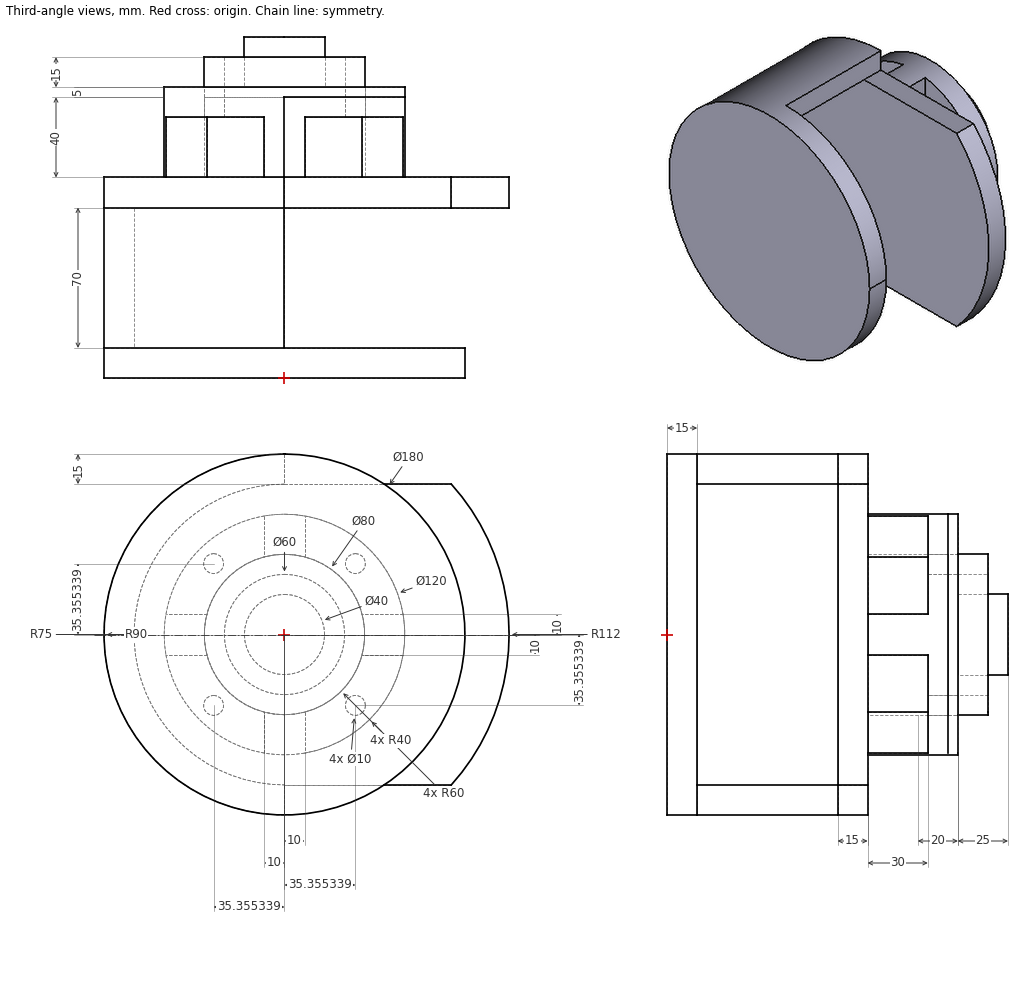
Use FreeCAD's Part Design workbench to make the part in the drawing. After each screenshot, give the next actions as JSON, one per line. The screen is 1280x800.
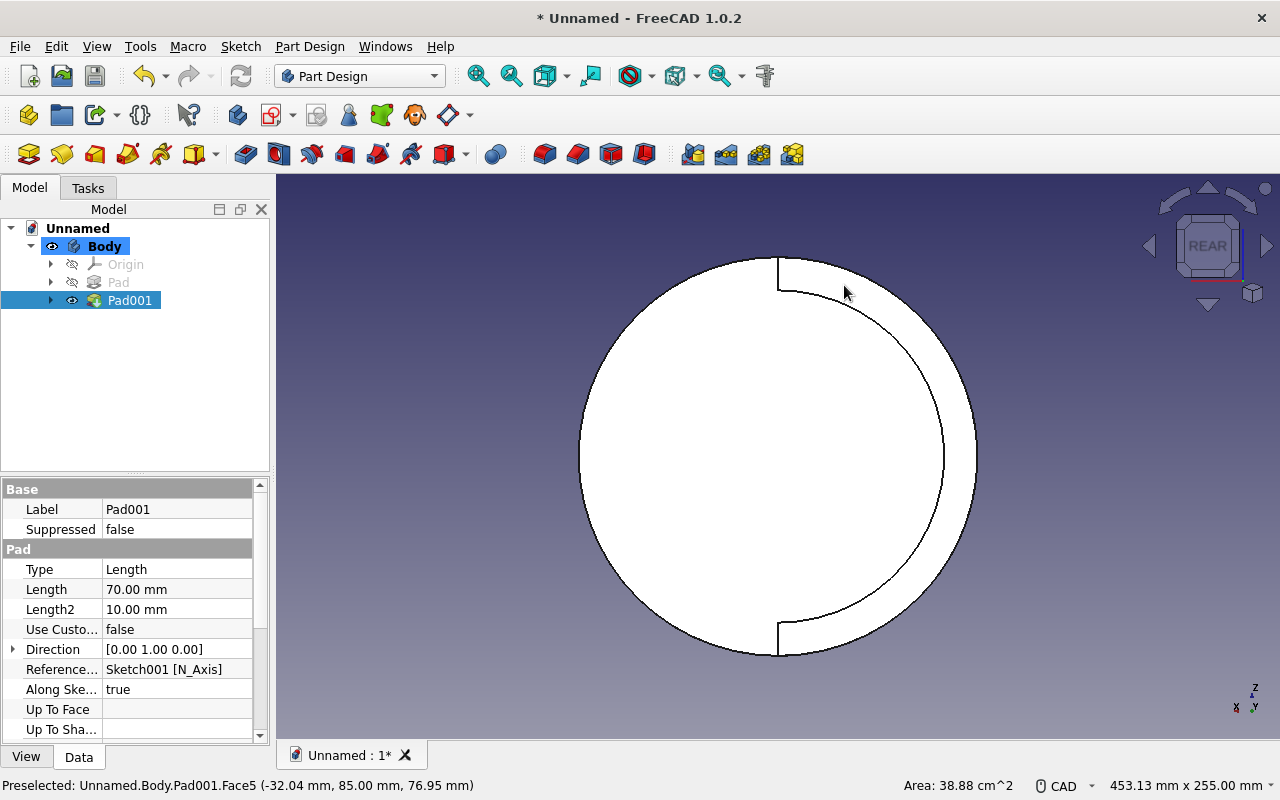
{"action": "left_click", "coordinate": [270, 116]}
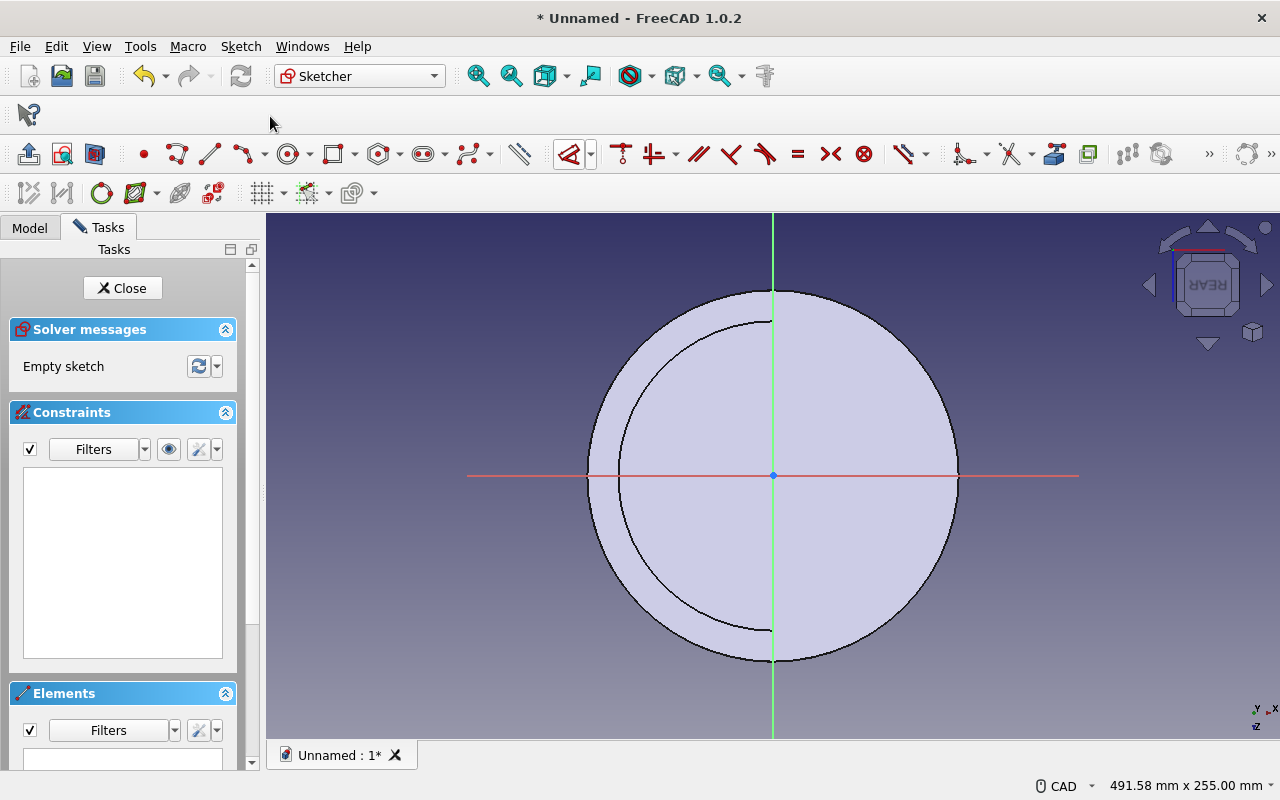
{"action": "key", "text": "g m"}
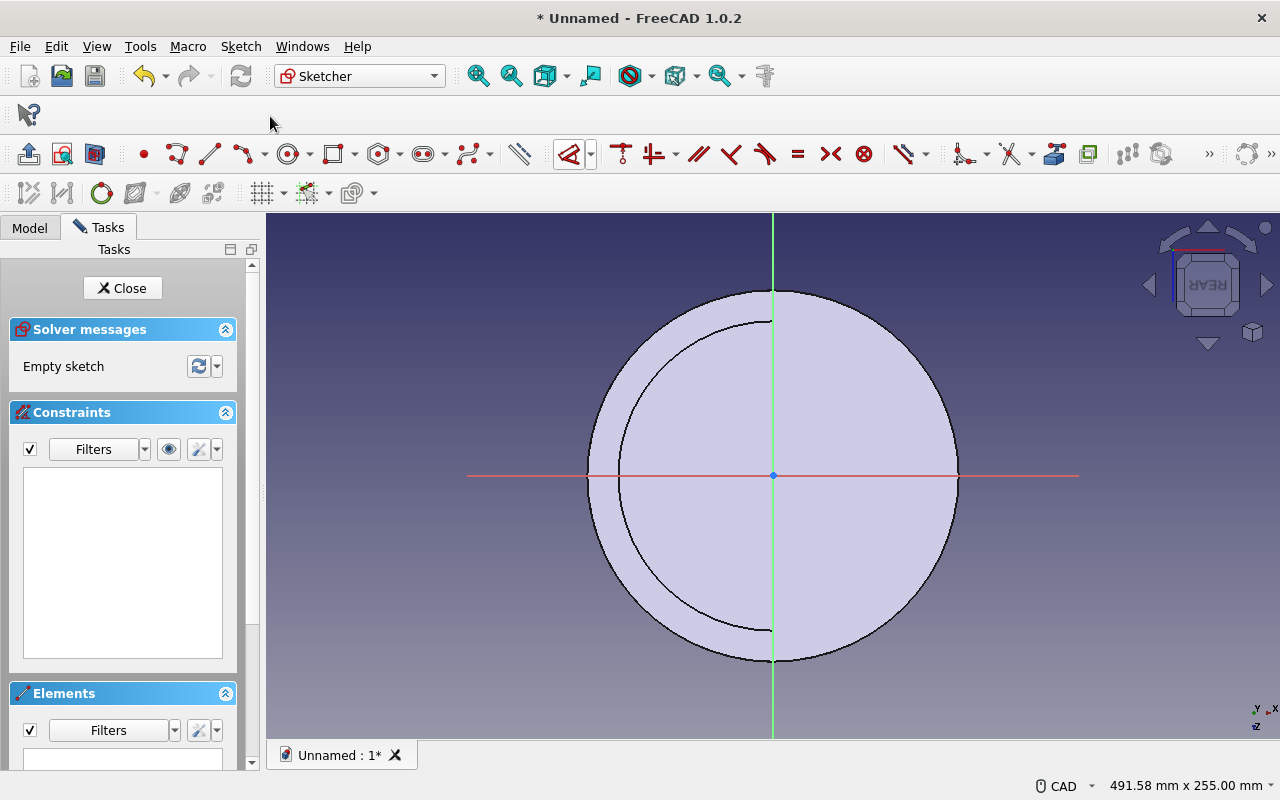
{"action": "left_click", "coordinate": [773, 662]}
{"action": "left_click", "coordinate": [782, 631]}
{"action": "left_click", "coordinate": [945, 631]}
{"action": "right_click", "coordinate": [945, 631]}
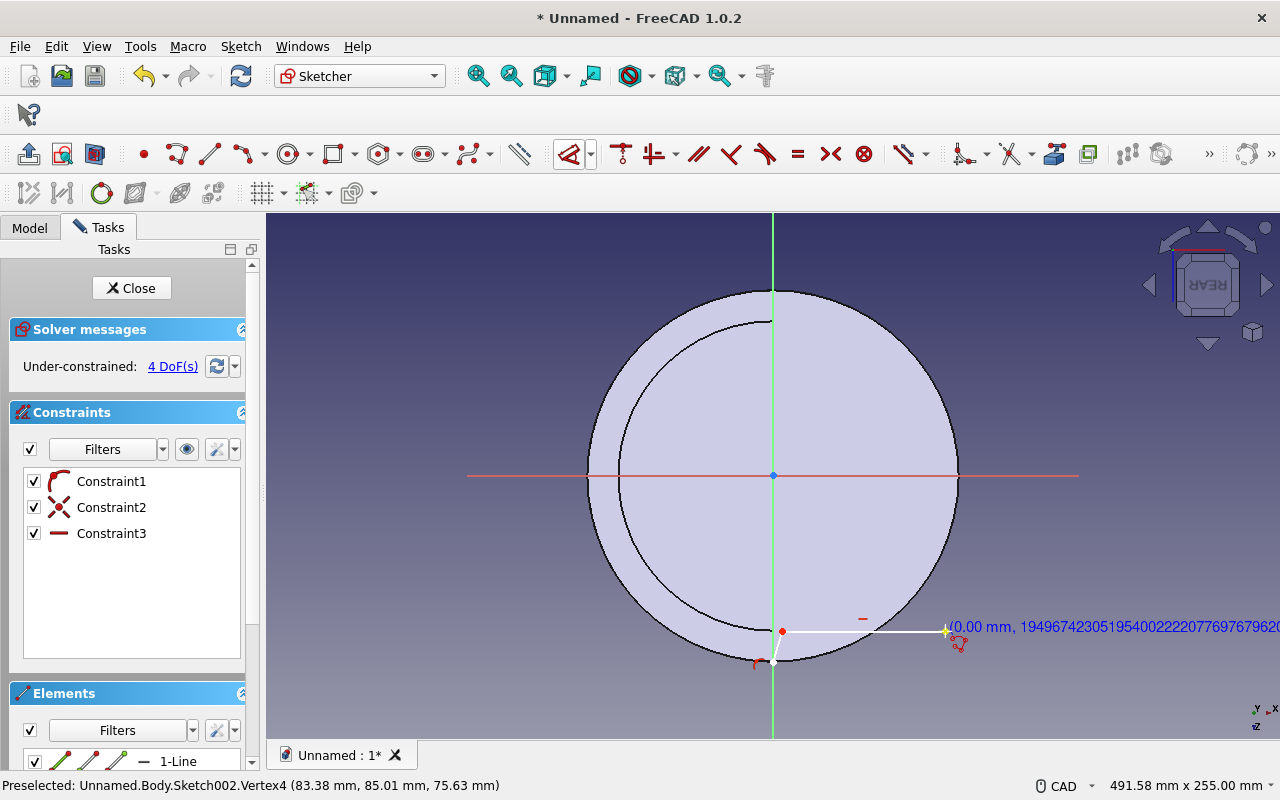
{"action": "left_click", "coordinate": [945, 321]}
{"action": "left_click", "coordinate": [773, 321]}
{"action": "left_click", "coordinate": [782, 290]}
{"action": "right_click", "coordinate": [782, 290]}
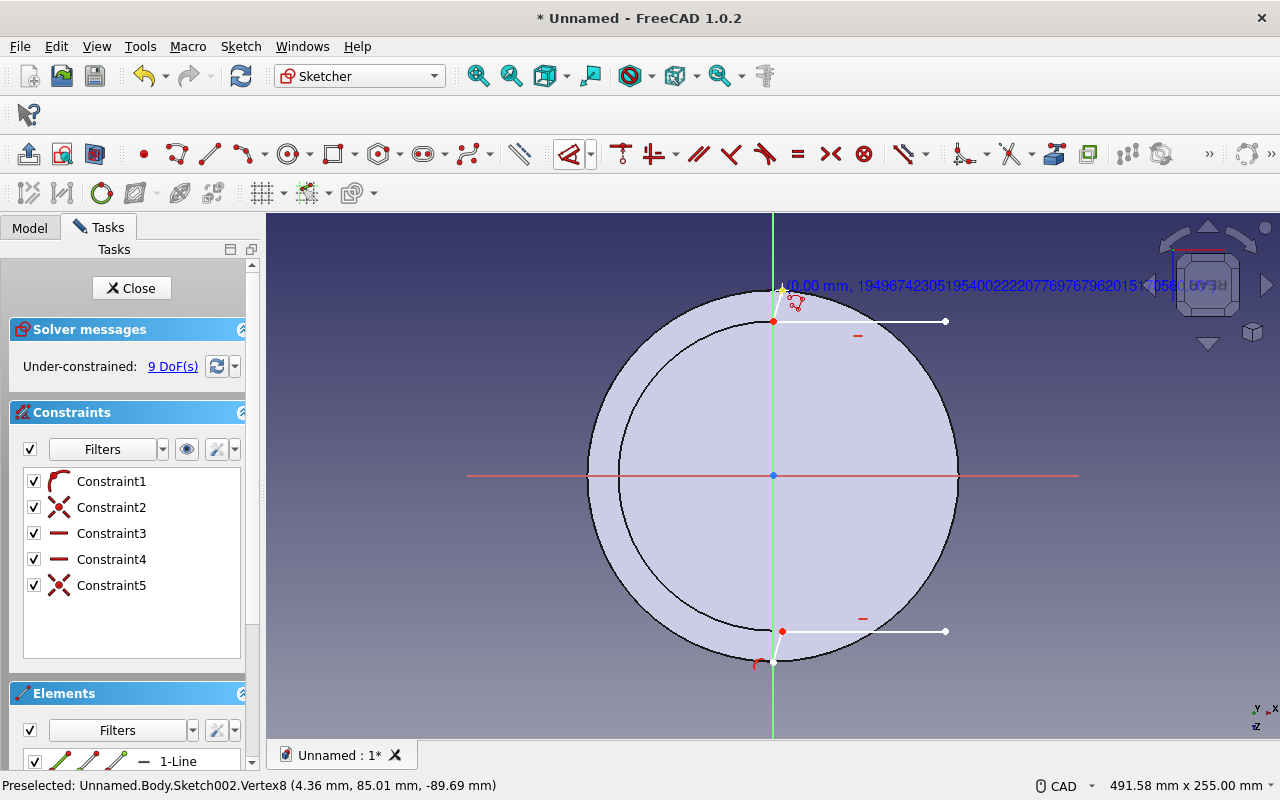
{"action": "left_click", "coordinate": [242, 154]}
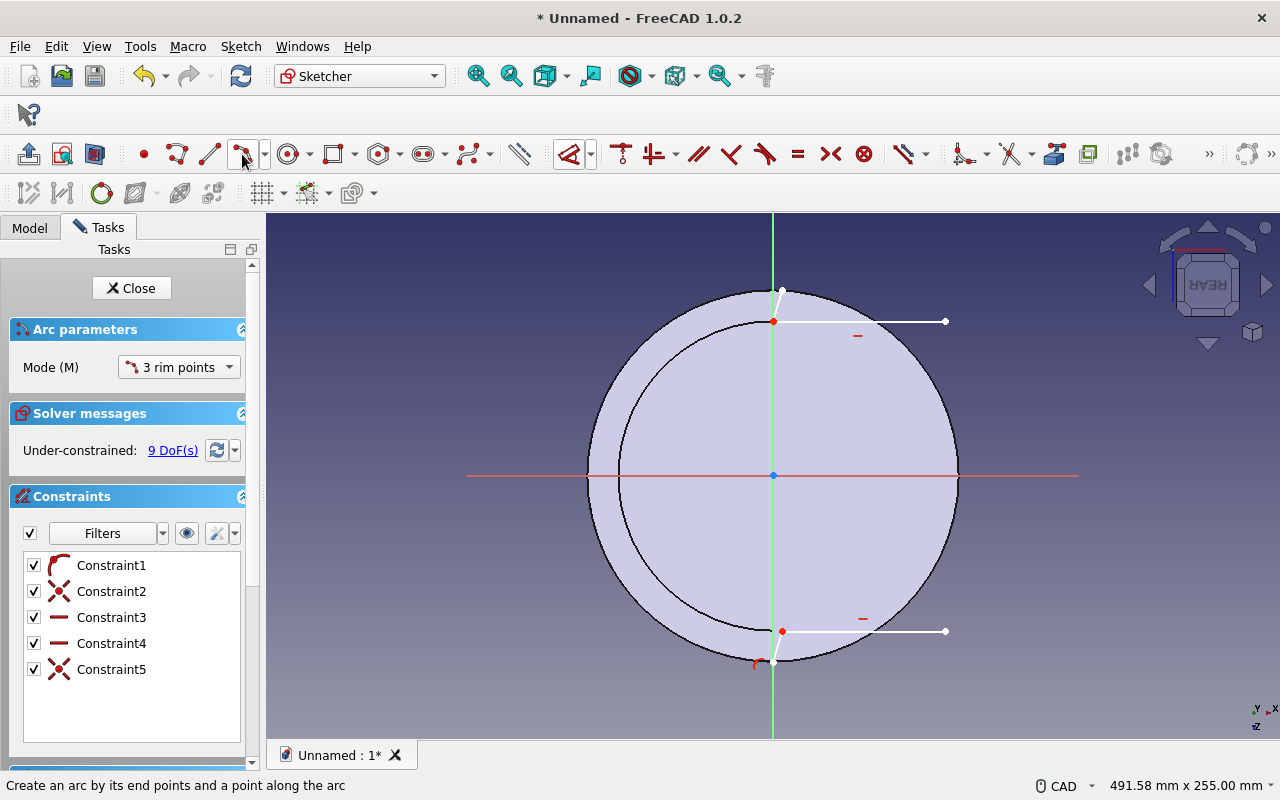
{"action": "left_click", "coordinate": [945, 632]}
{"action": "left_click", "coordinate": [945, 322]}
{"action": "left_click", "coordinate": [1002, 510]}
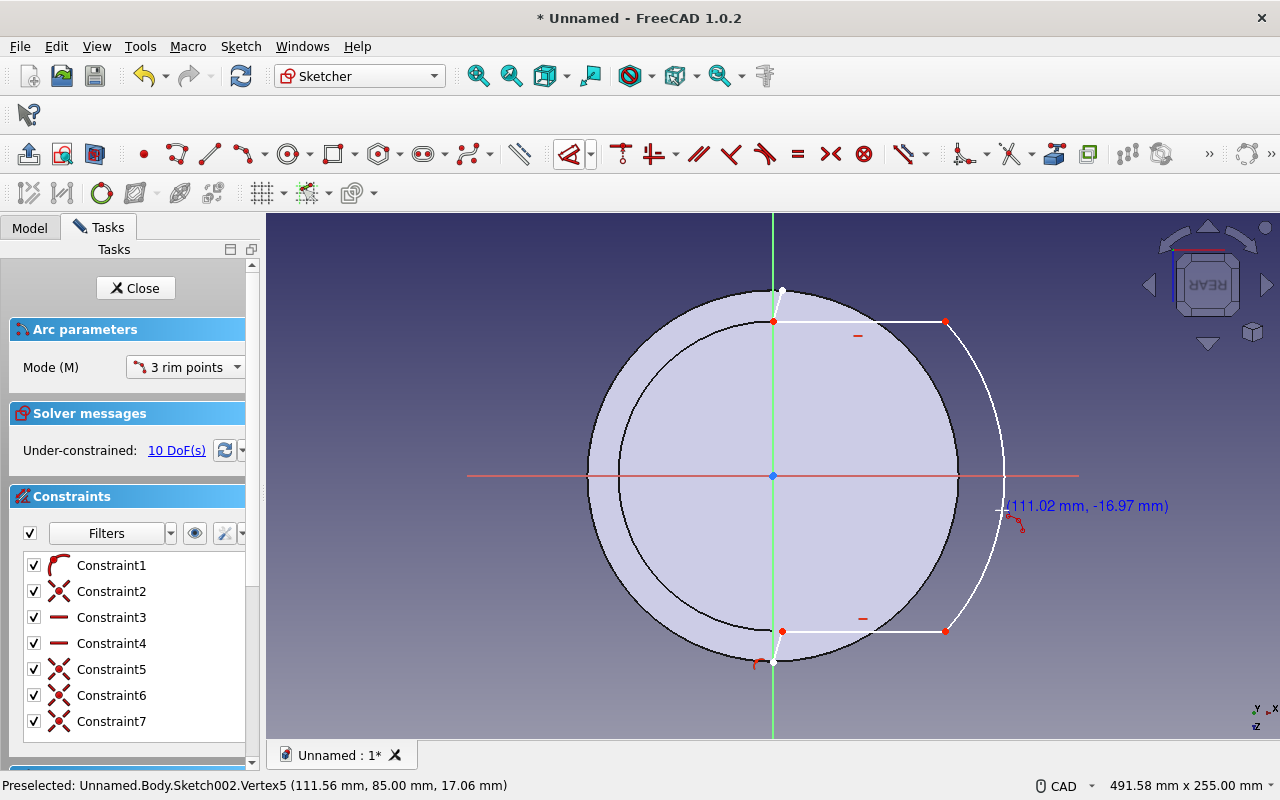
{"action": "left_click", "coordinate": [782, 291]}
{"action": "left_click", "coordinate": [773, 663]}
{"action": "left_click", "coordinate": [596, 419]}
{"action": "key", "text": "Escape"}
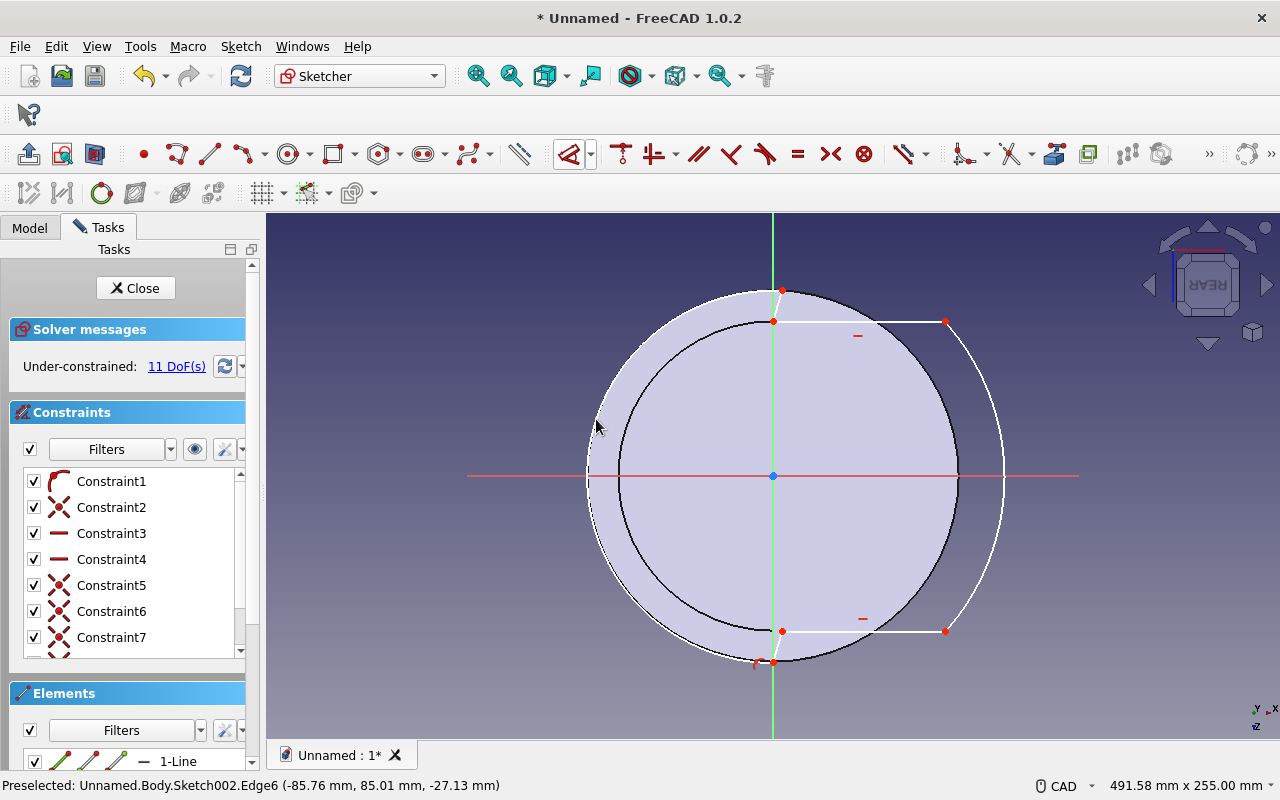
{"action": "scroll", "coordinate": [776, 654], "scroll_direction": "up", "scroll_amount": 2}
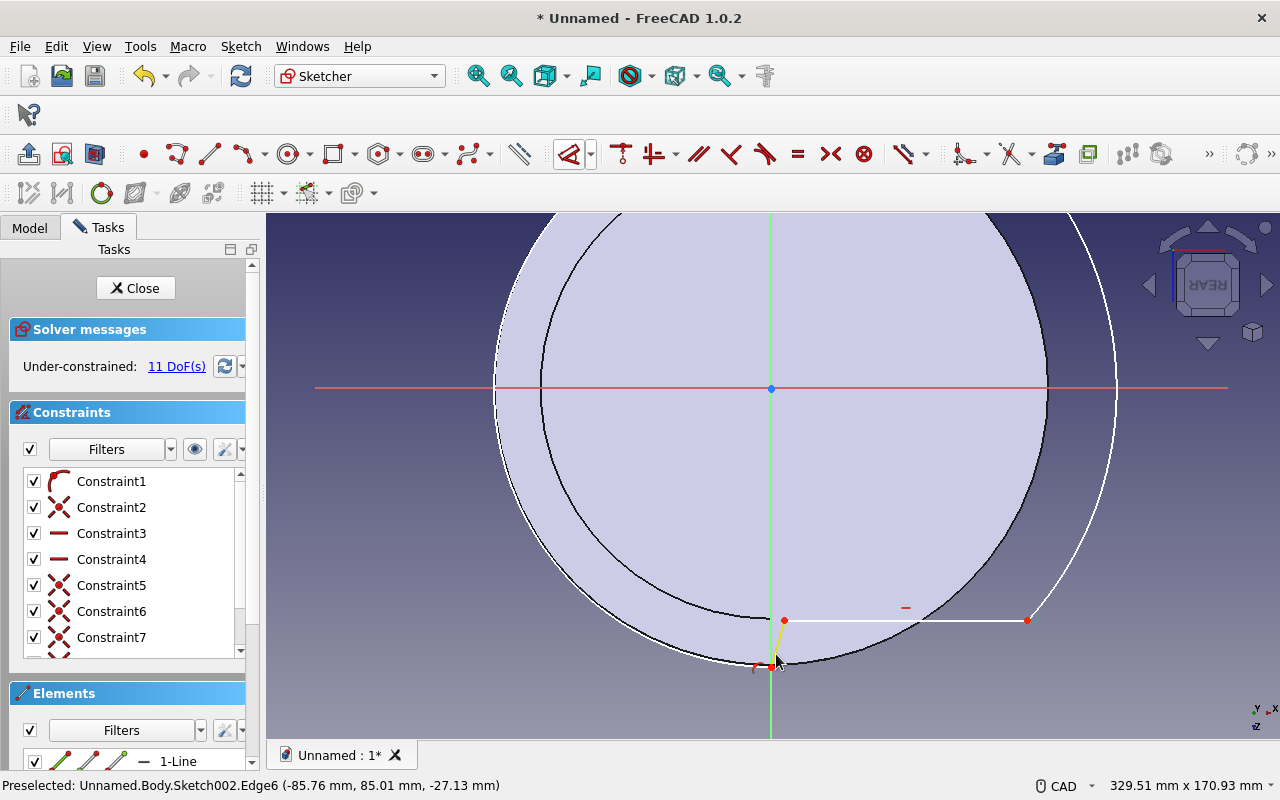
{"action": "left_click", "coordinate": [775, 653]}